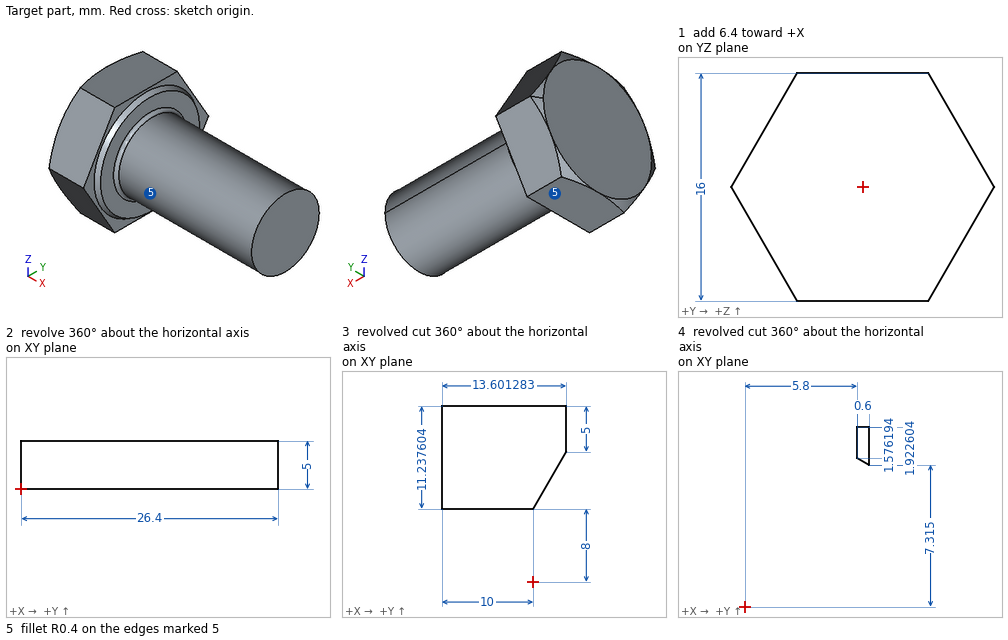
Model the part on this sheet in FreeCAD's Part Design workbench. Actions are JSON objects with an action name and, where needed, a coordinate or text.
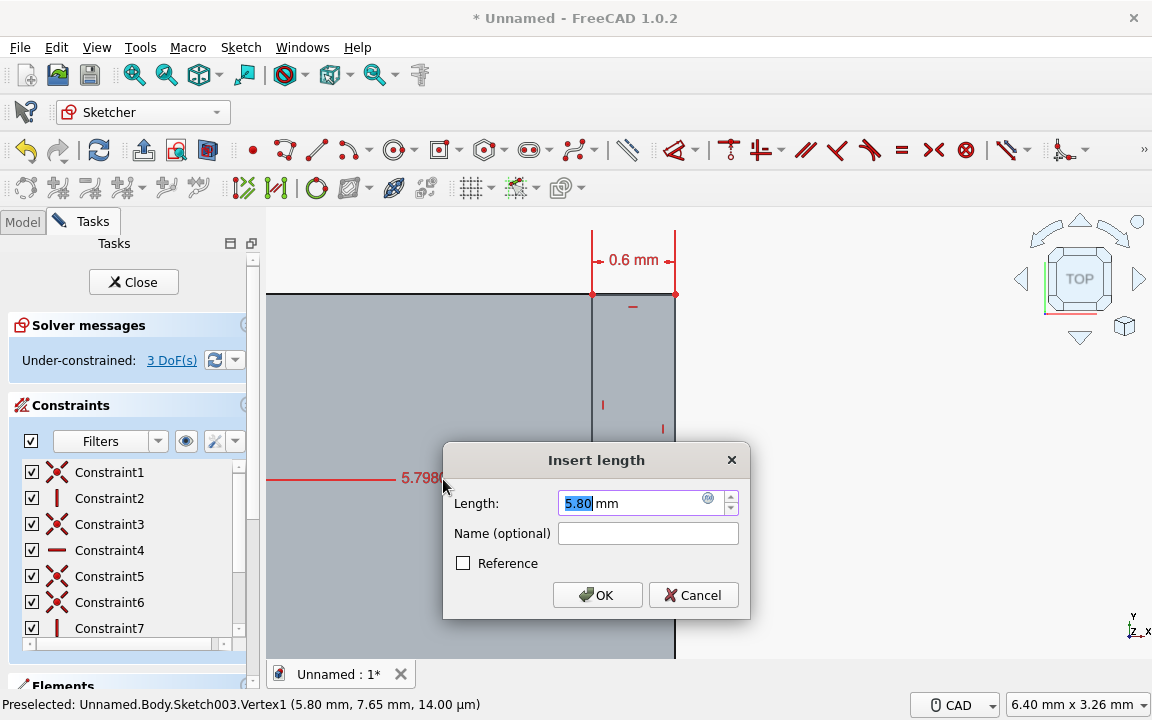
{"action": "type", "text": "5.8"}
{"action": "key", "text": "Return"}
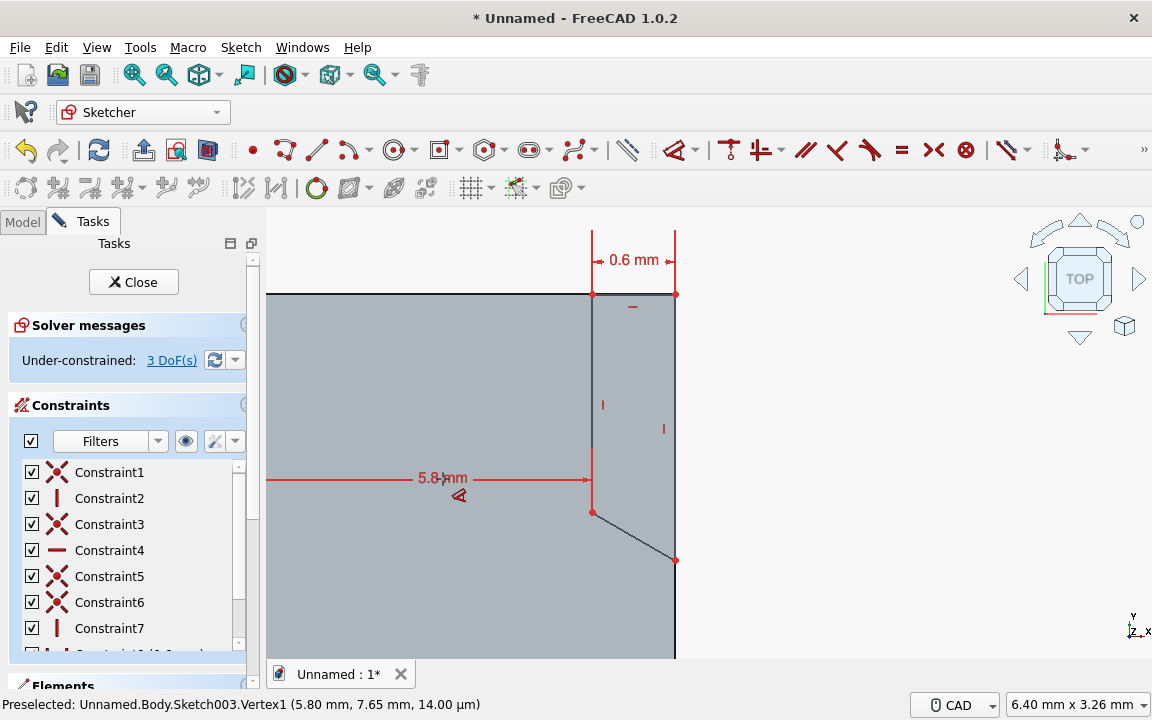
{"action": "left_click", "coordinate": [675, 561]}
{"action": "left_click", "coordinate": [709, 596]}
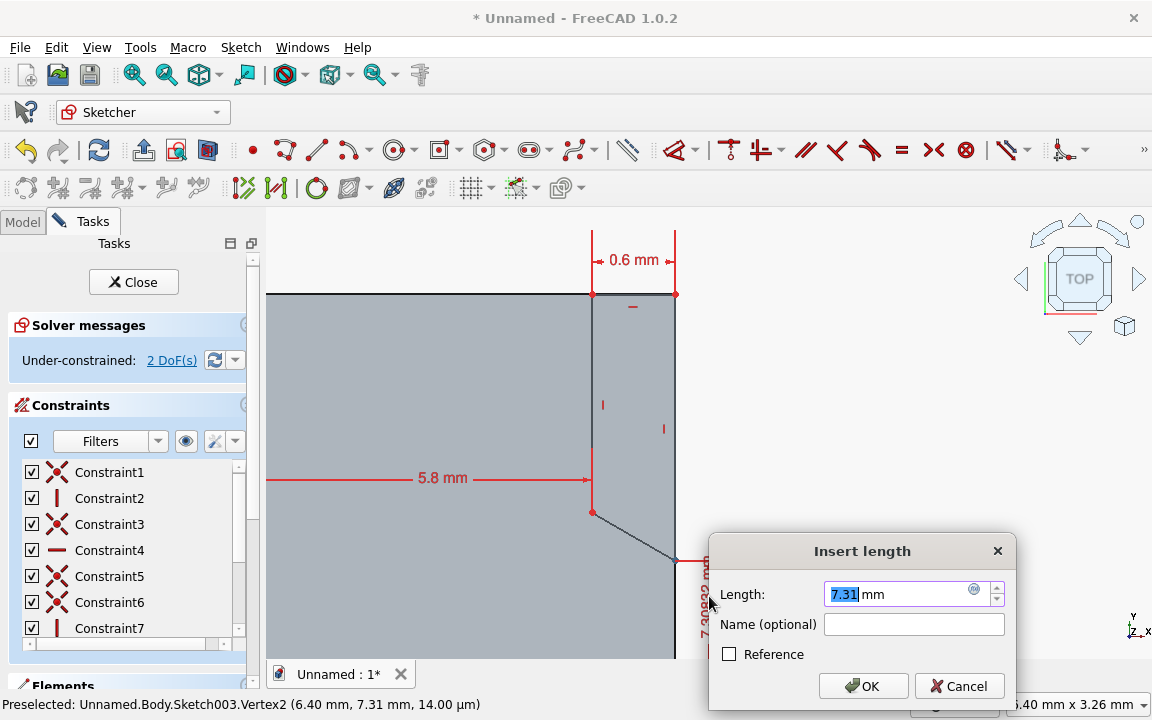
{"action": "type", "text": "7.315"}
{"action": "key", "text": "Return"}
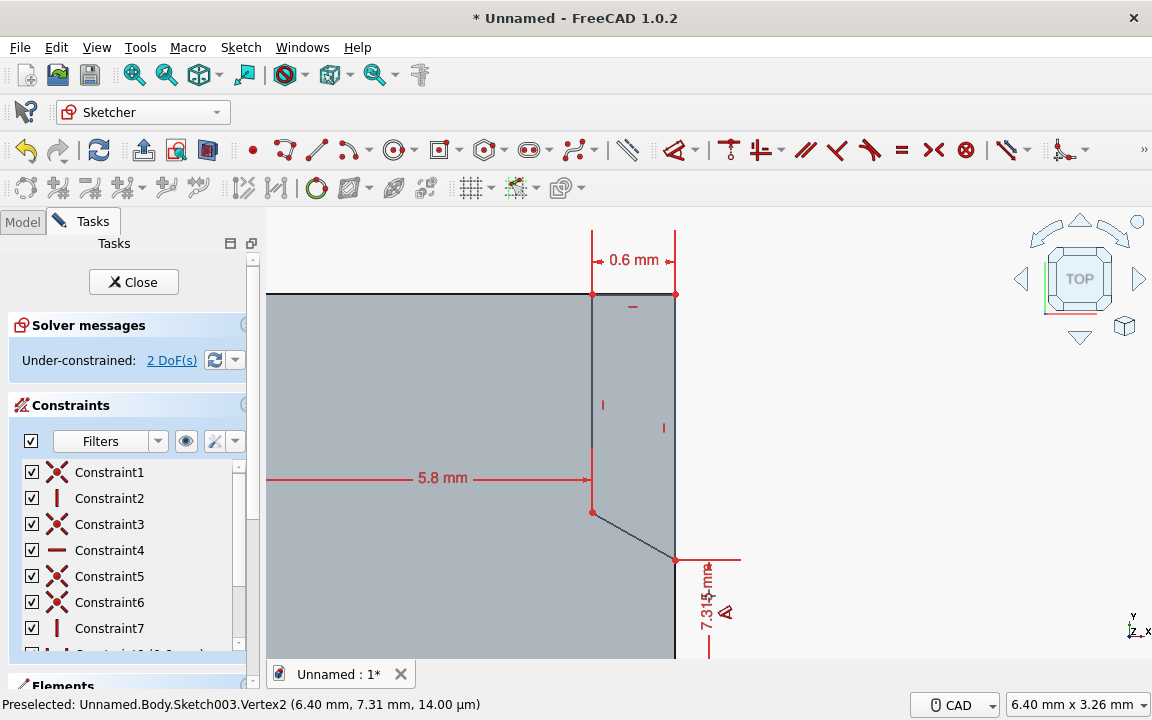
{"action": "left_click", "coordinate": [675, 481]}
{"action": "left_click", "coordinate": [709, 428]}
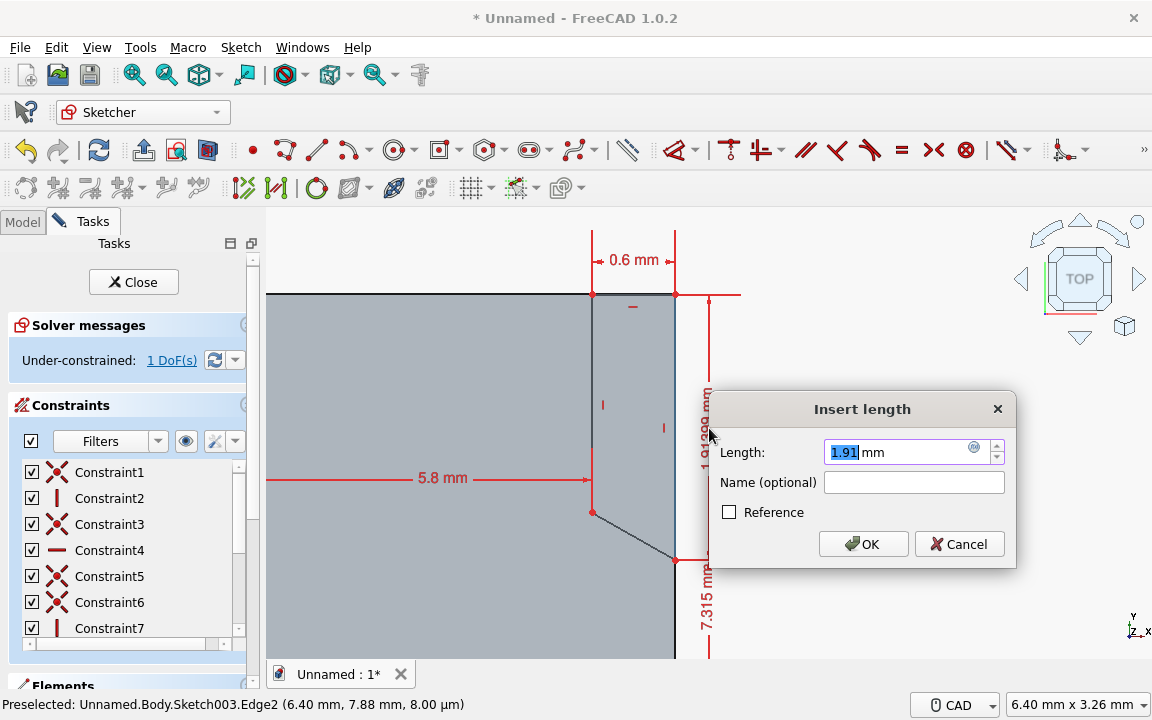
{"action": "type", "text": "1.922604"}
{"action": "key", "text": "Return"}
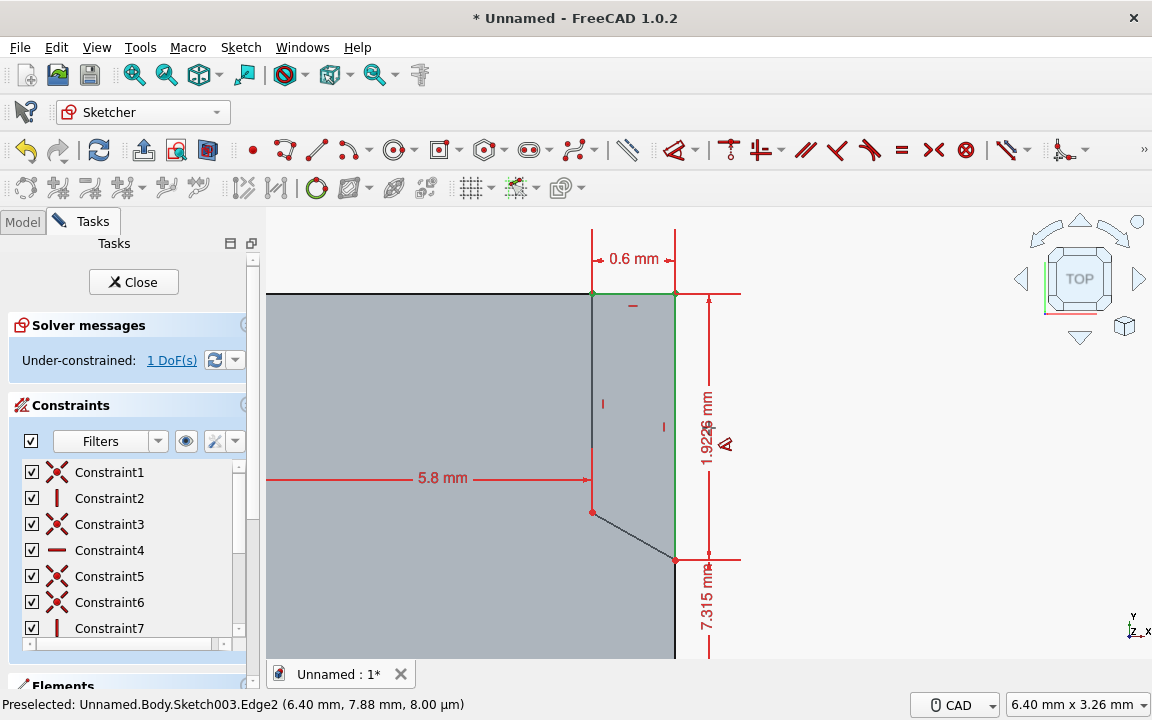
{"action": "left_click", "coordinate": [592, 360]}
{"action": "left_click", "coordinate": [558, 403]}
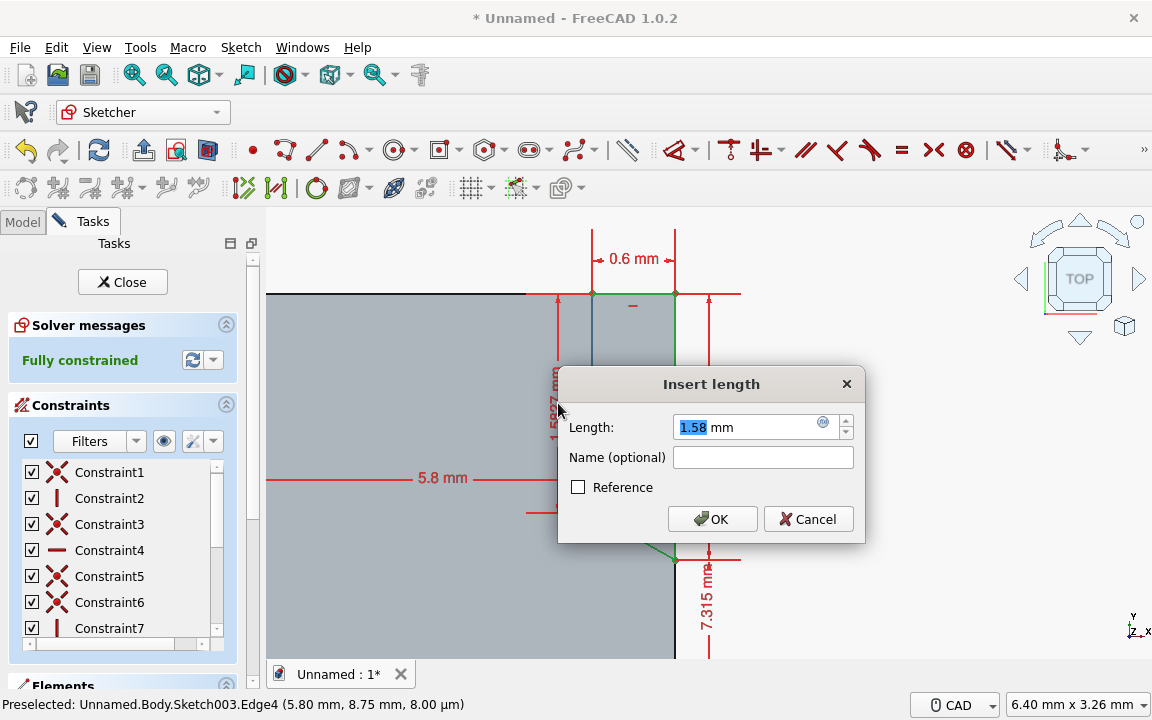
{"action": "type", "text": "1.576194"}
{"action": "key", "text": "Return"}
{"action": "key", "text": "Escape"}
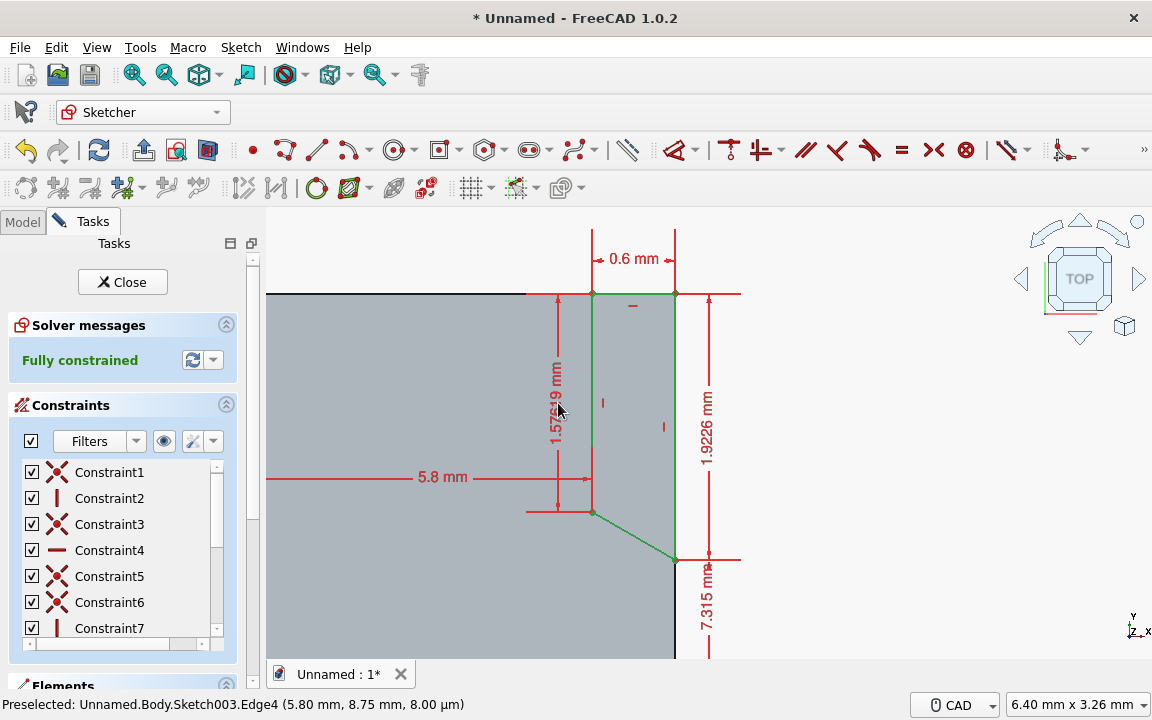
{"action": "left_click", "coordinate": [123, 282]}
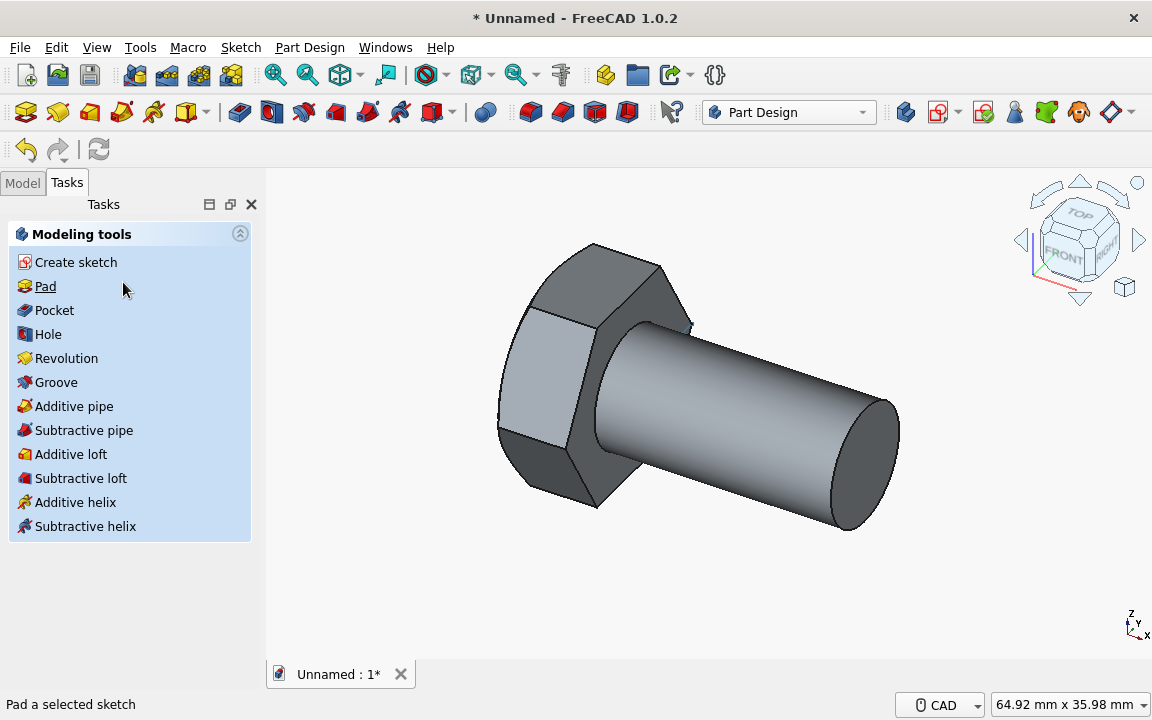
{"action": "left_click", "coordinate": [304, 112]}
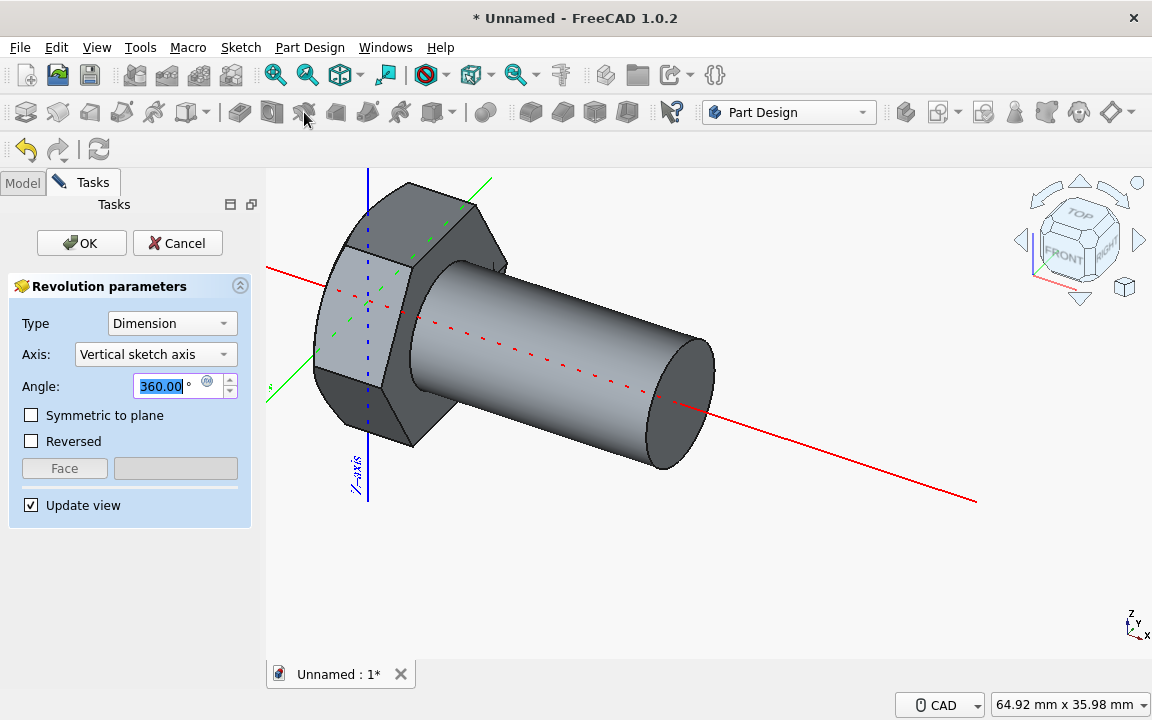
{"action": "left_click", "coordinate": [156, 354]}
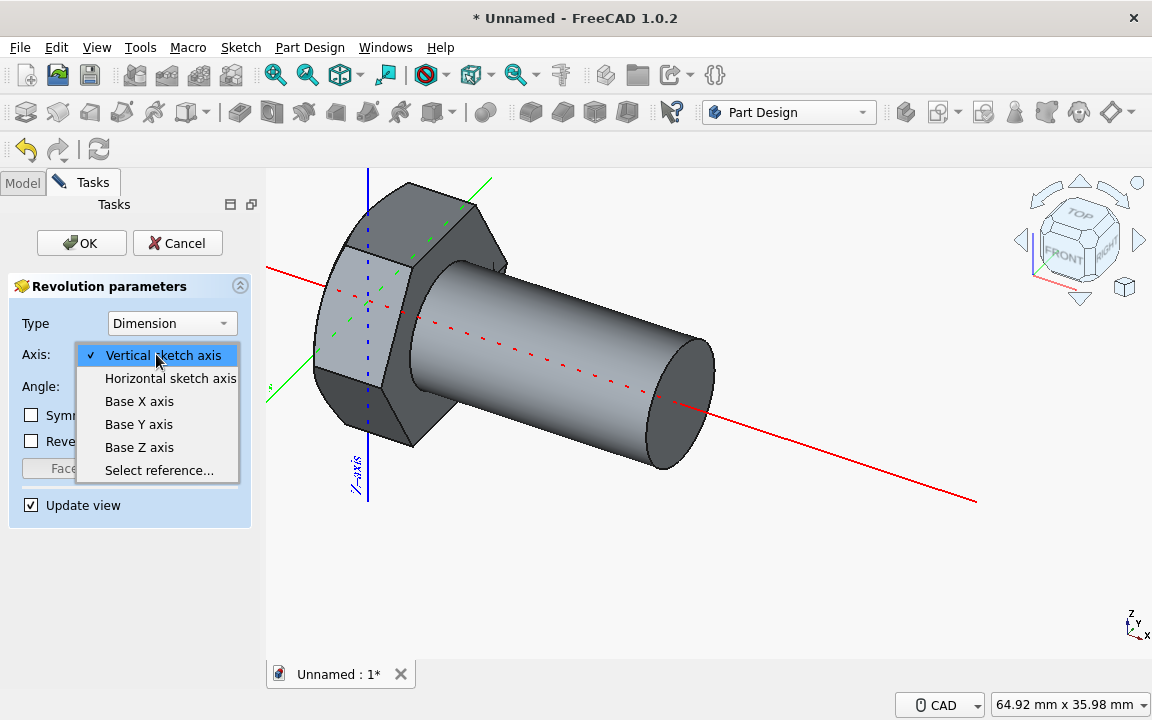
{"action": "left_click", "coordinate": [156, 378]}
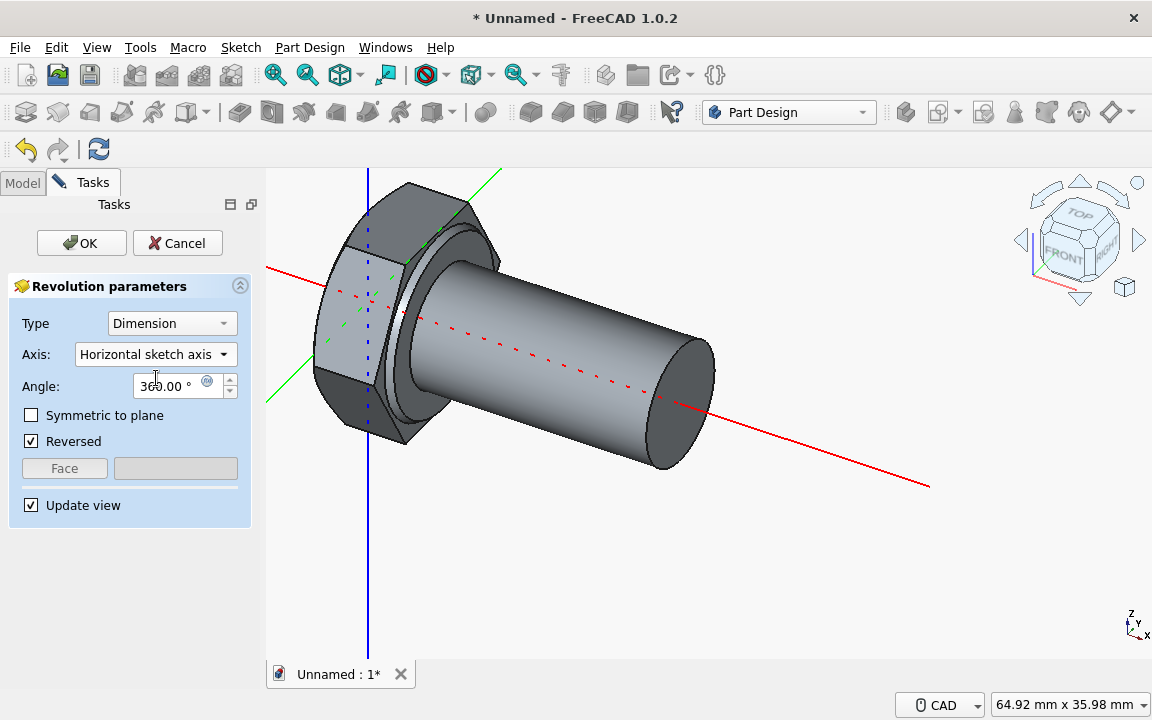
{"action": "left_click", "coordinate": [82, 243]}